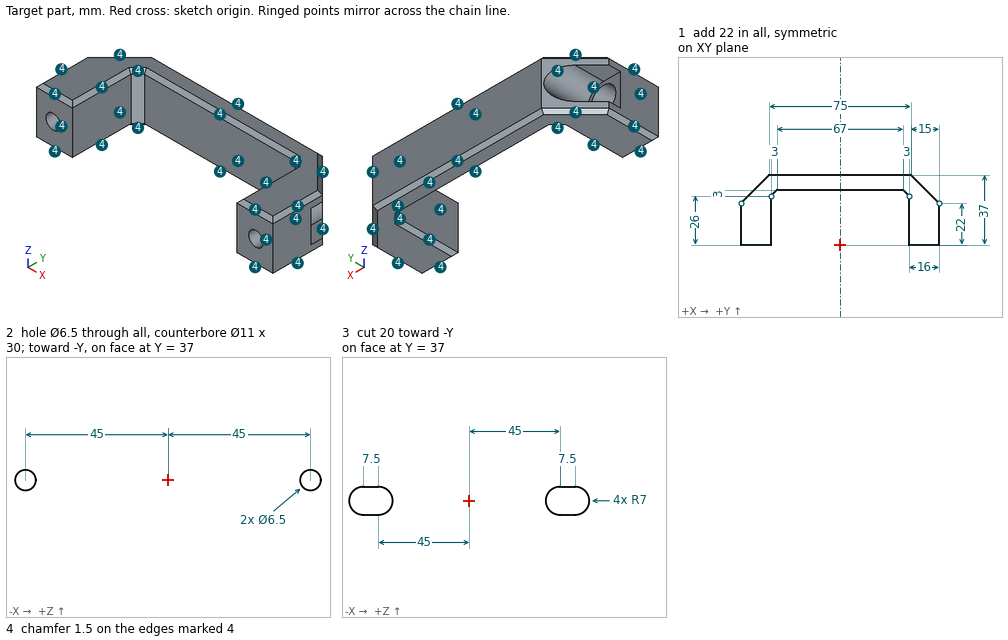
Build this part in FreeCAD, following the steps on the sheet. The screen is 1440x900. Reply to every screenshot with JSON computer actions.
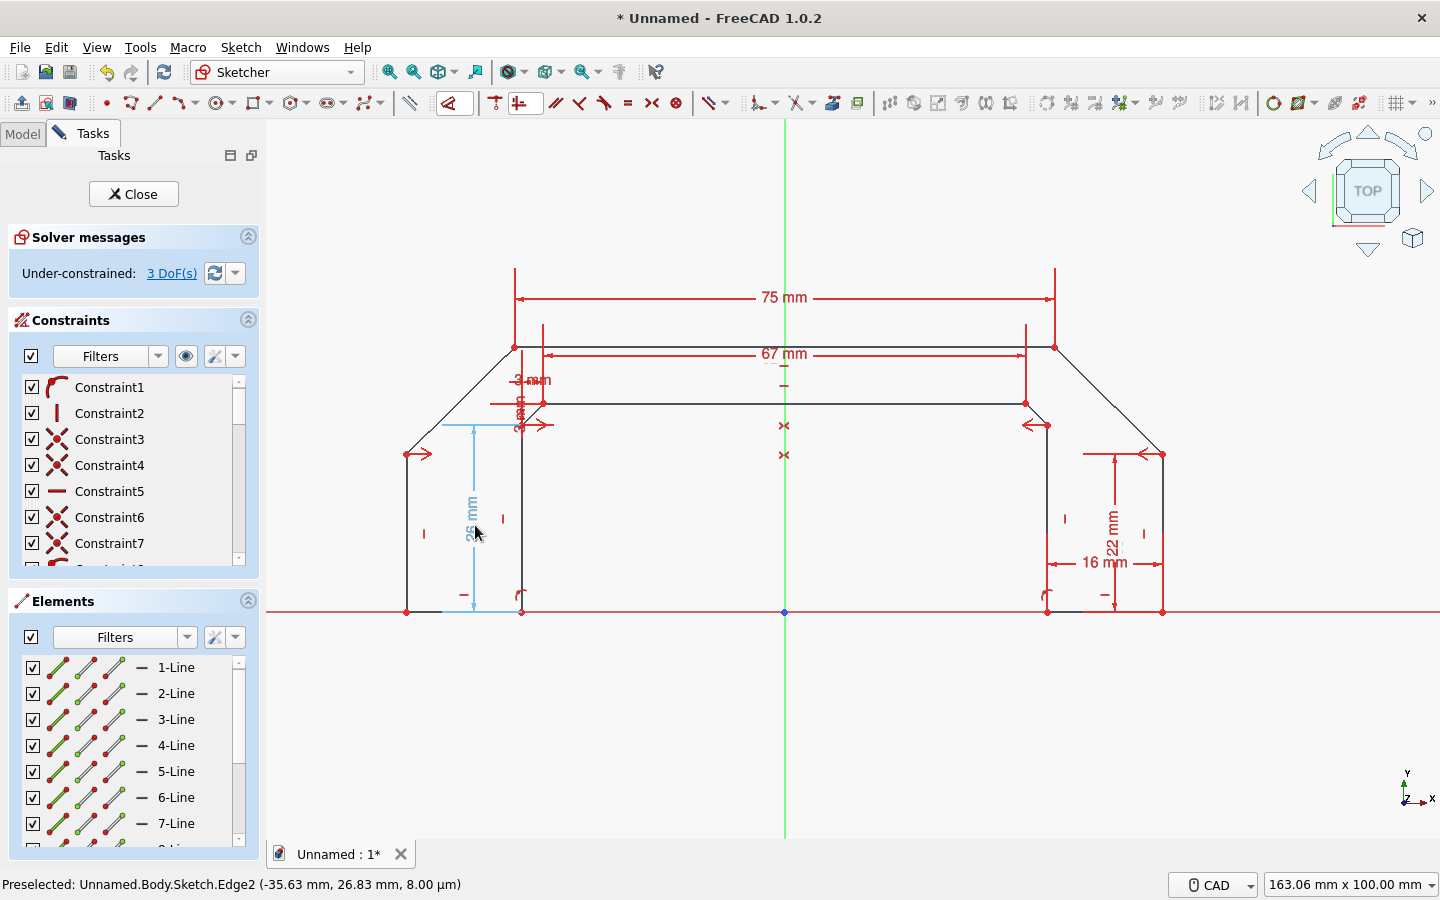
{"action": "scroll", "coordinate": [1032, 410], "scroll_direction": "up", "scroll_amount": 4}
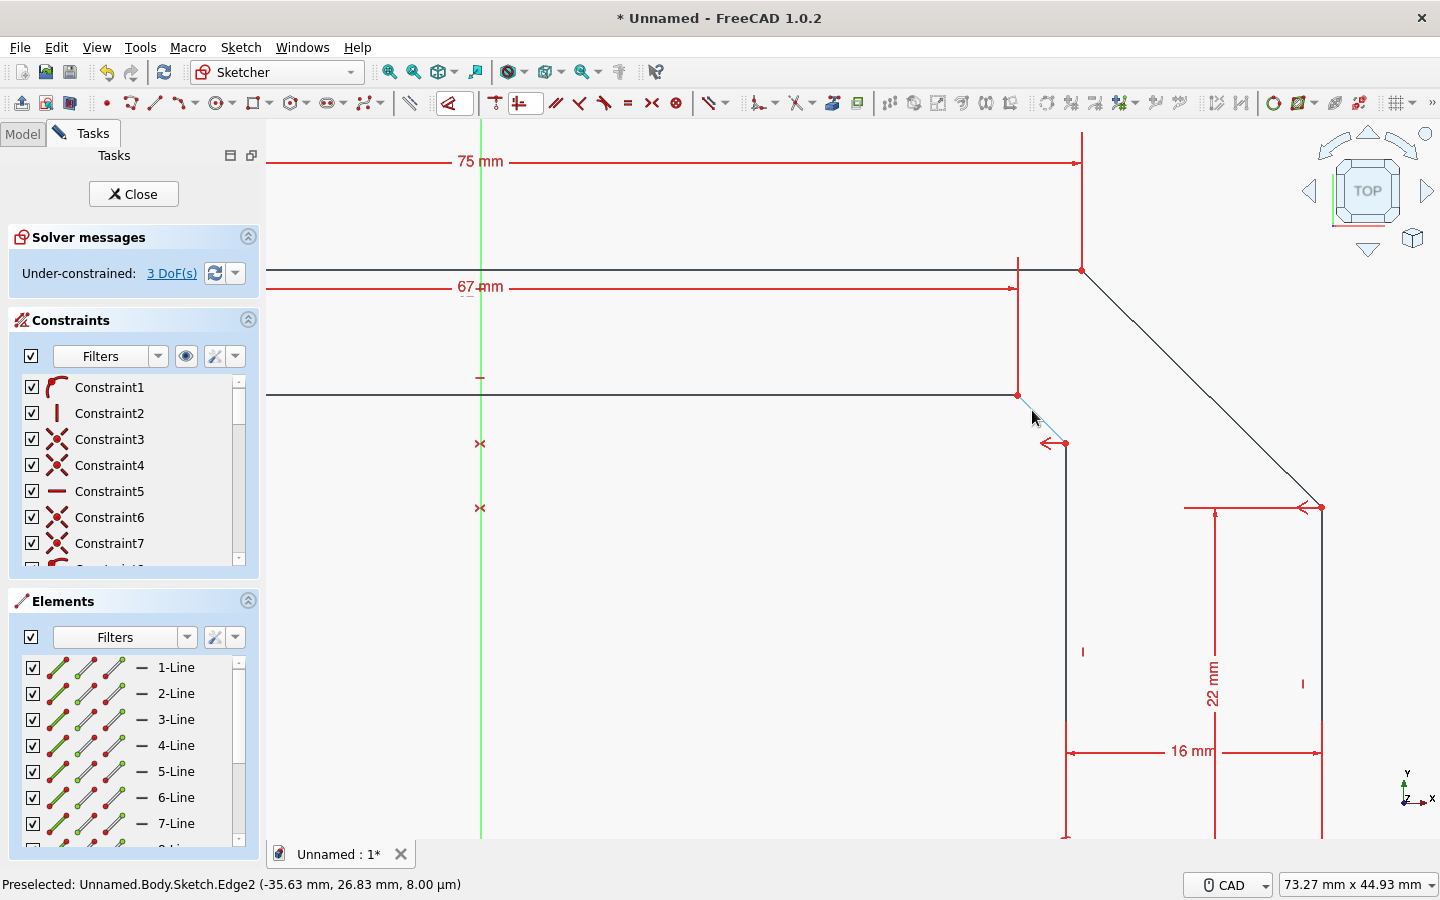
{"action": "left_click", "coordinate": [1032, 410]}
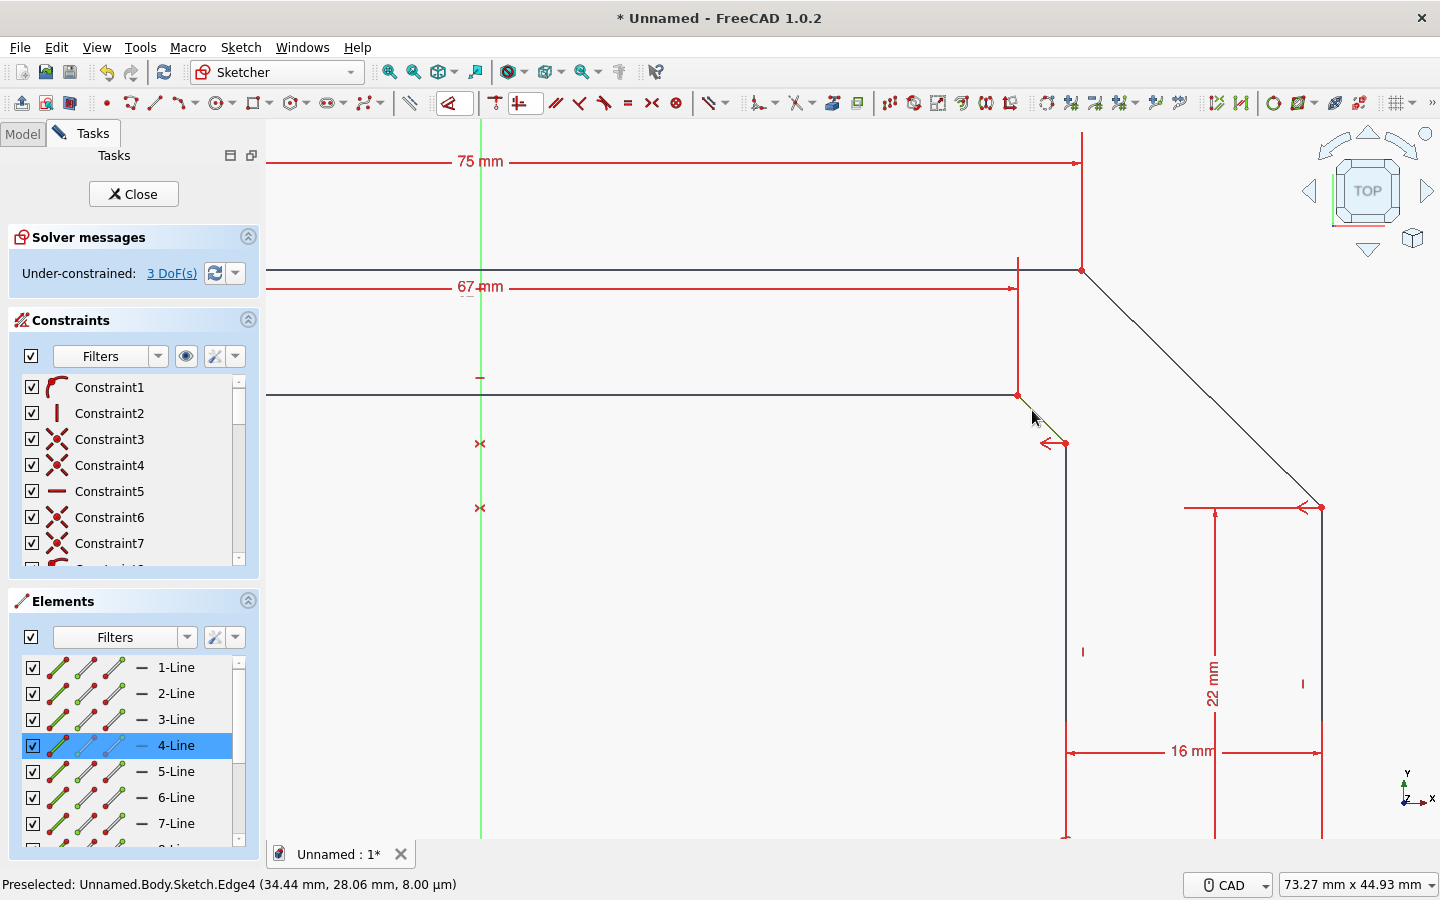
{"action": "key", "text": "l"}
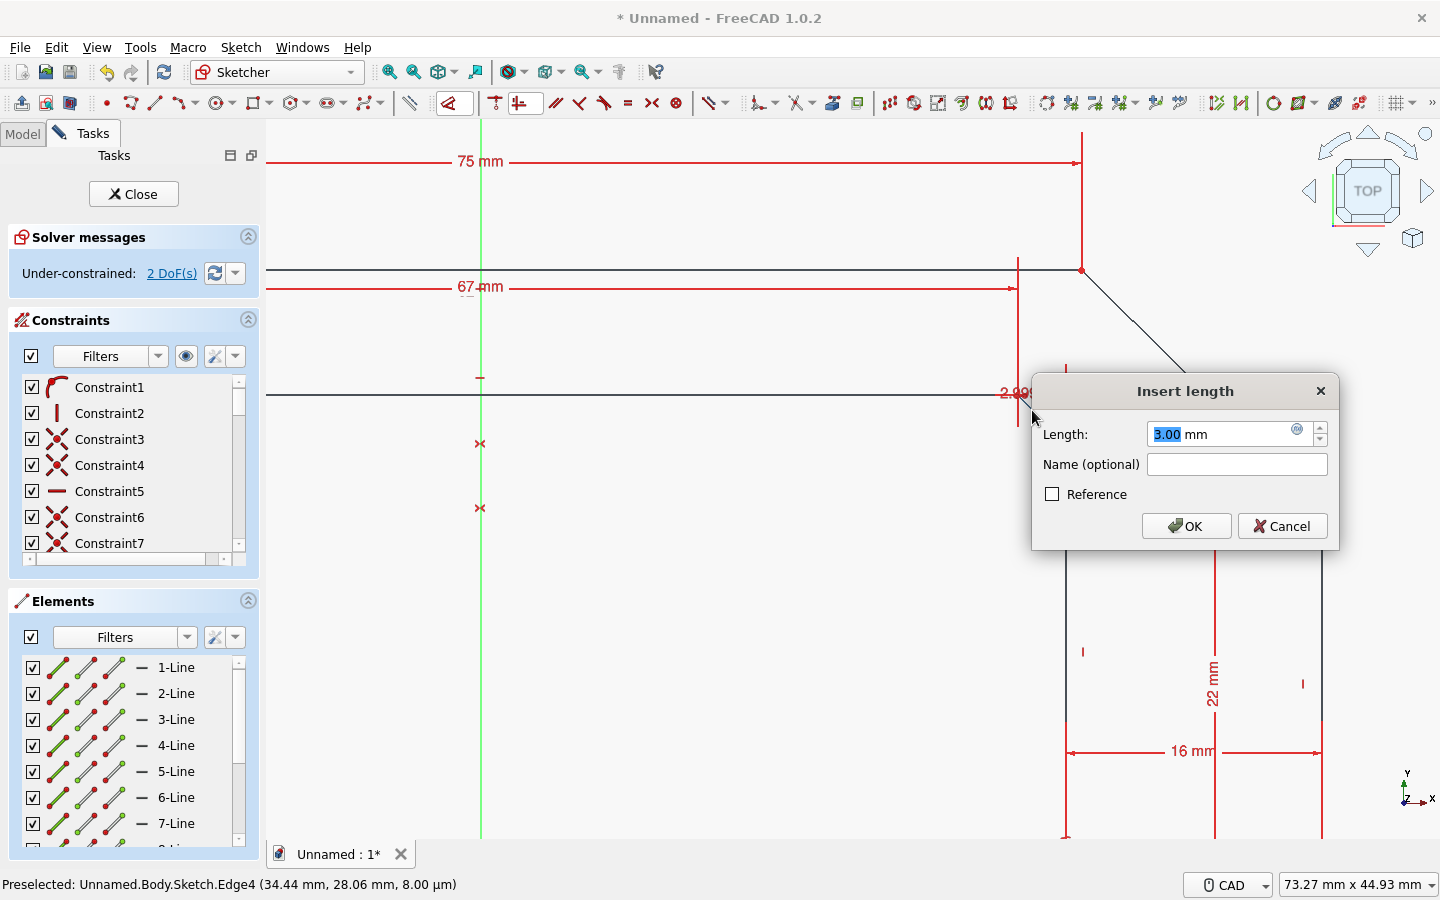
{"action": "type", "text": "3"}
{"action": "key", "text": "Return"}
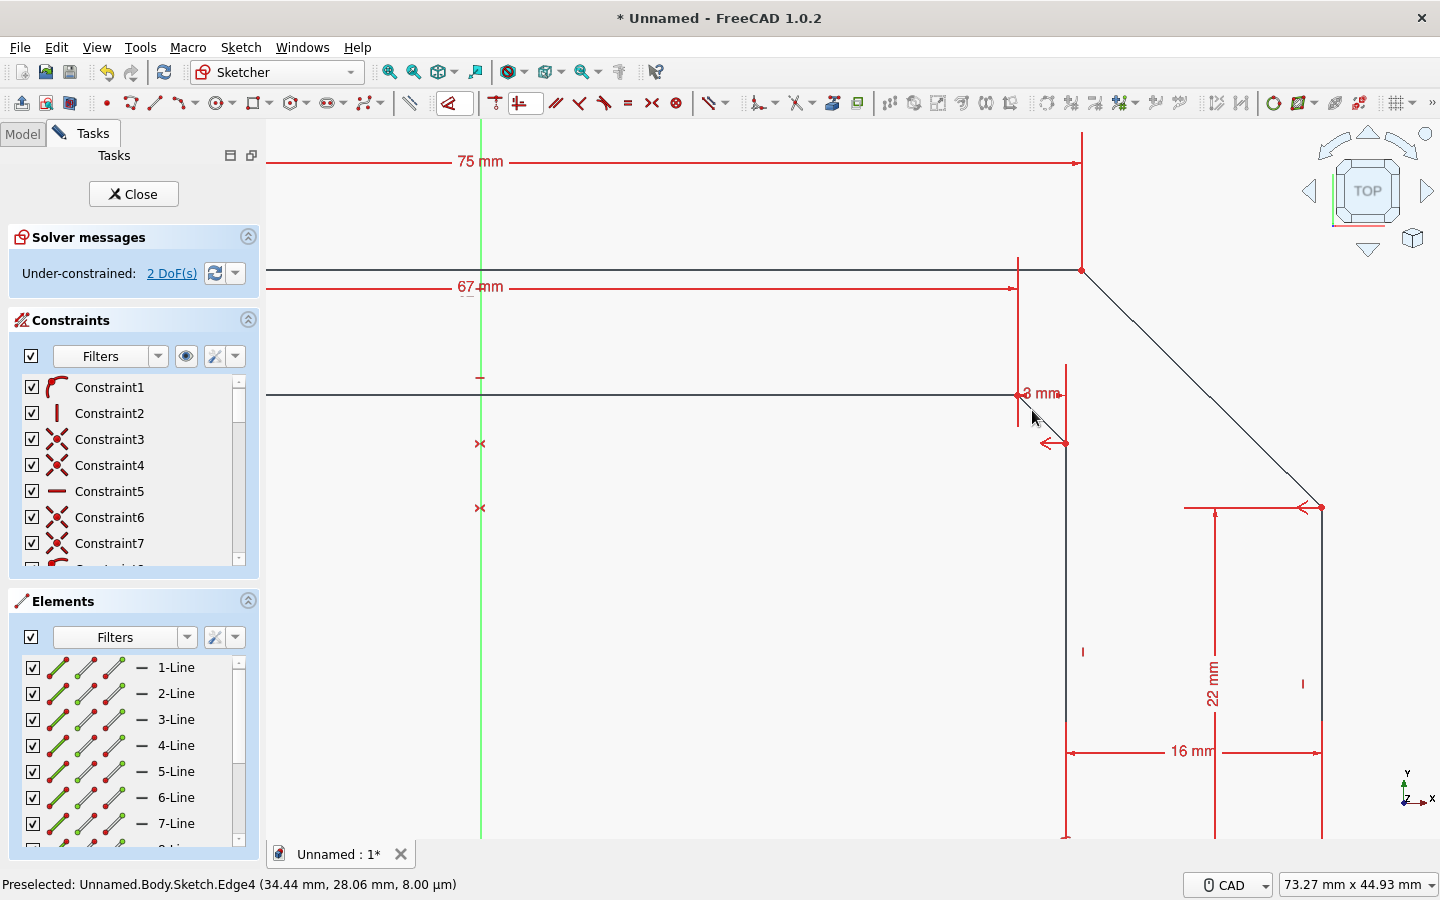
{"action": "left_click", "coordinate": [1082, 270]}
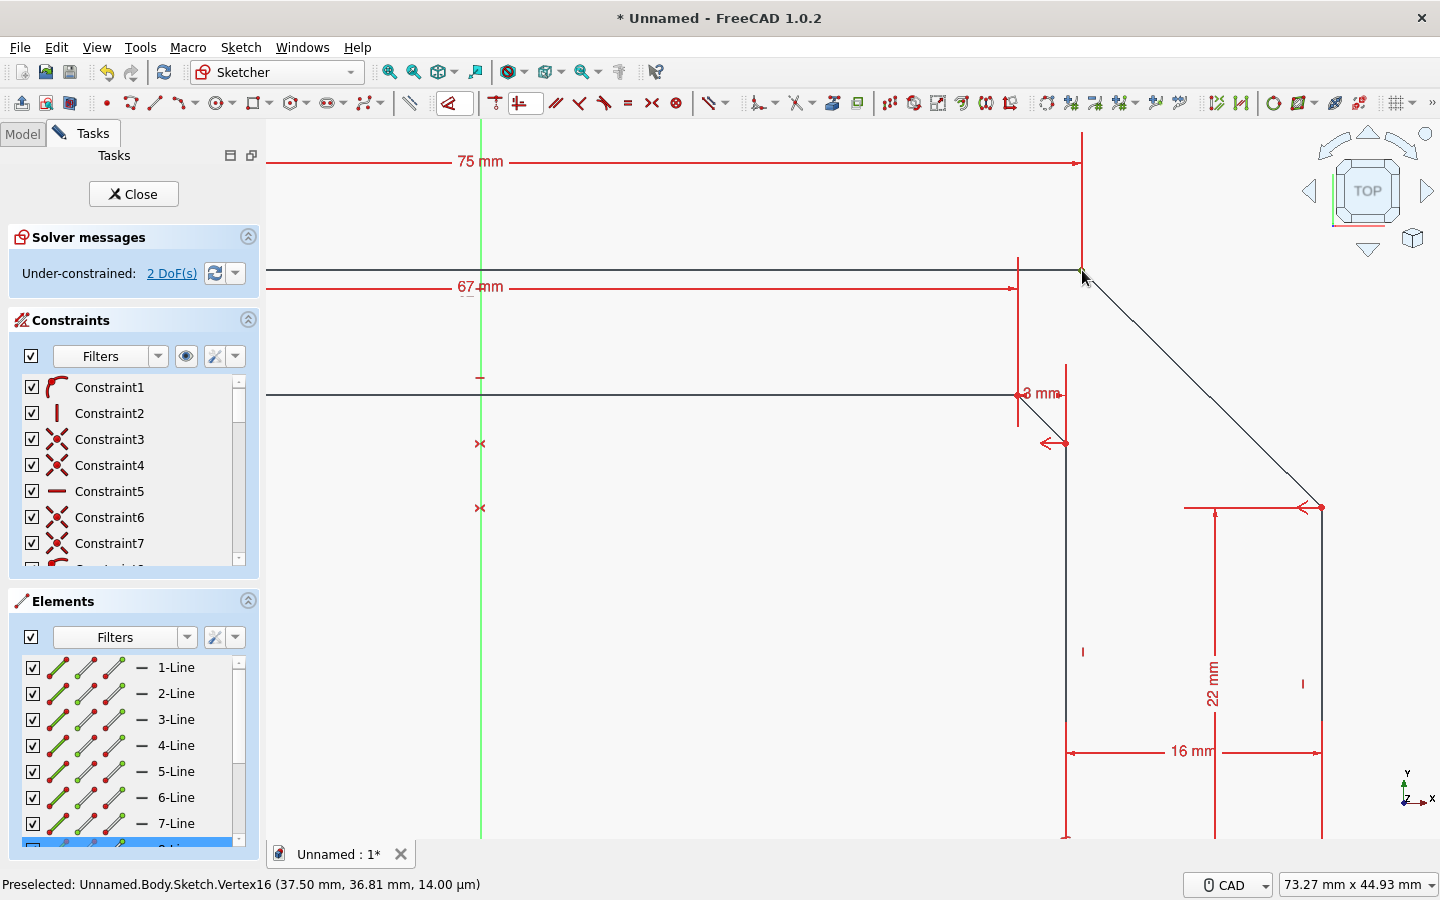
{"action": "key", "text": "i"}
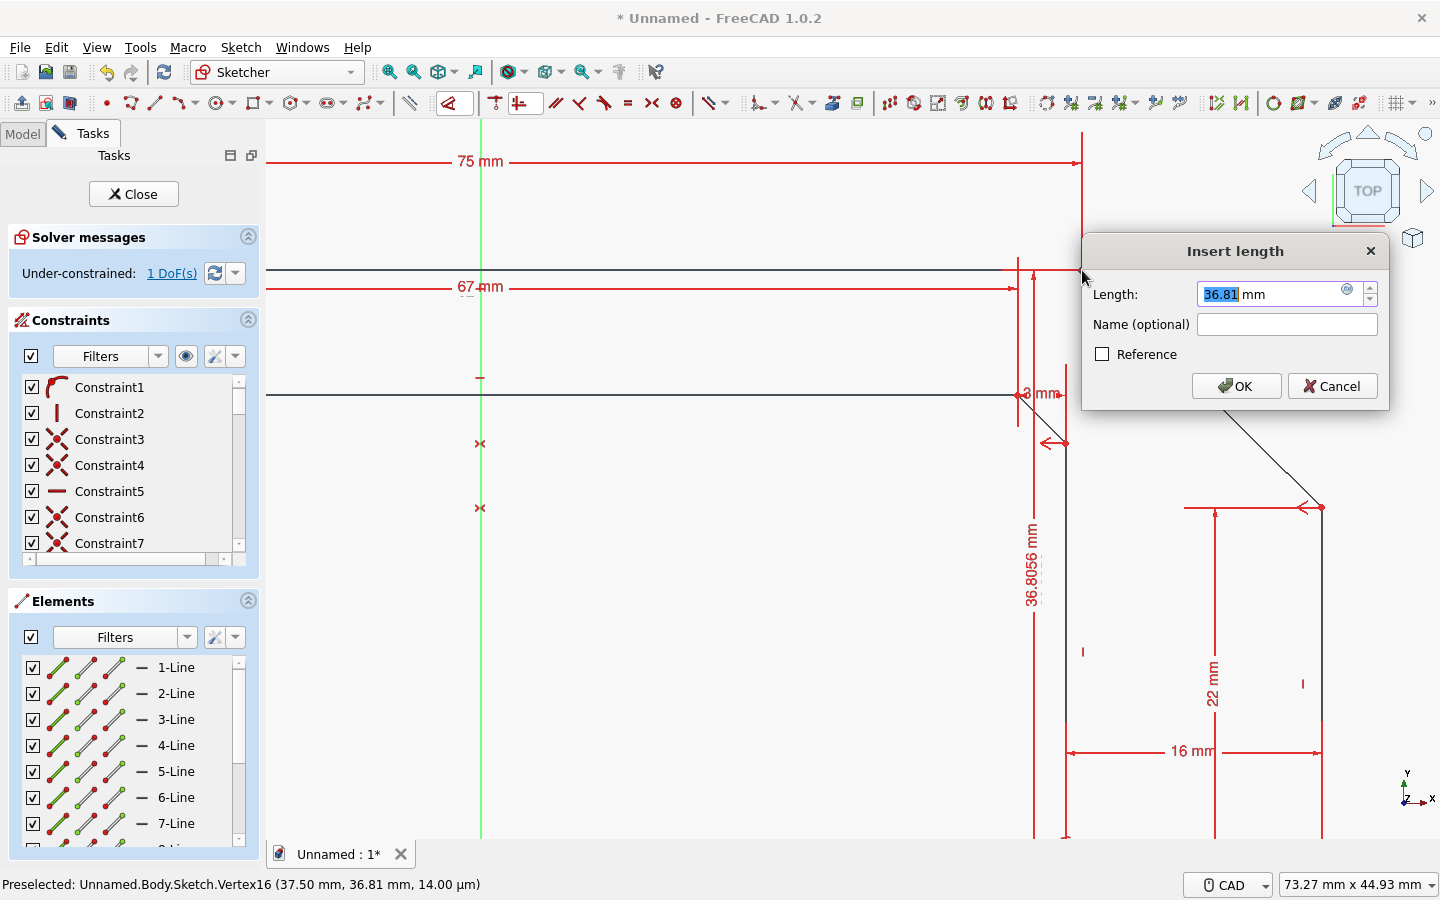
{"action": "type", "text": "37"}
{"action": "key", "text": "Return"}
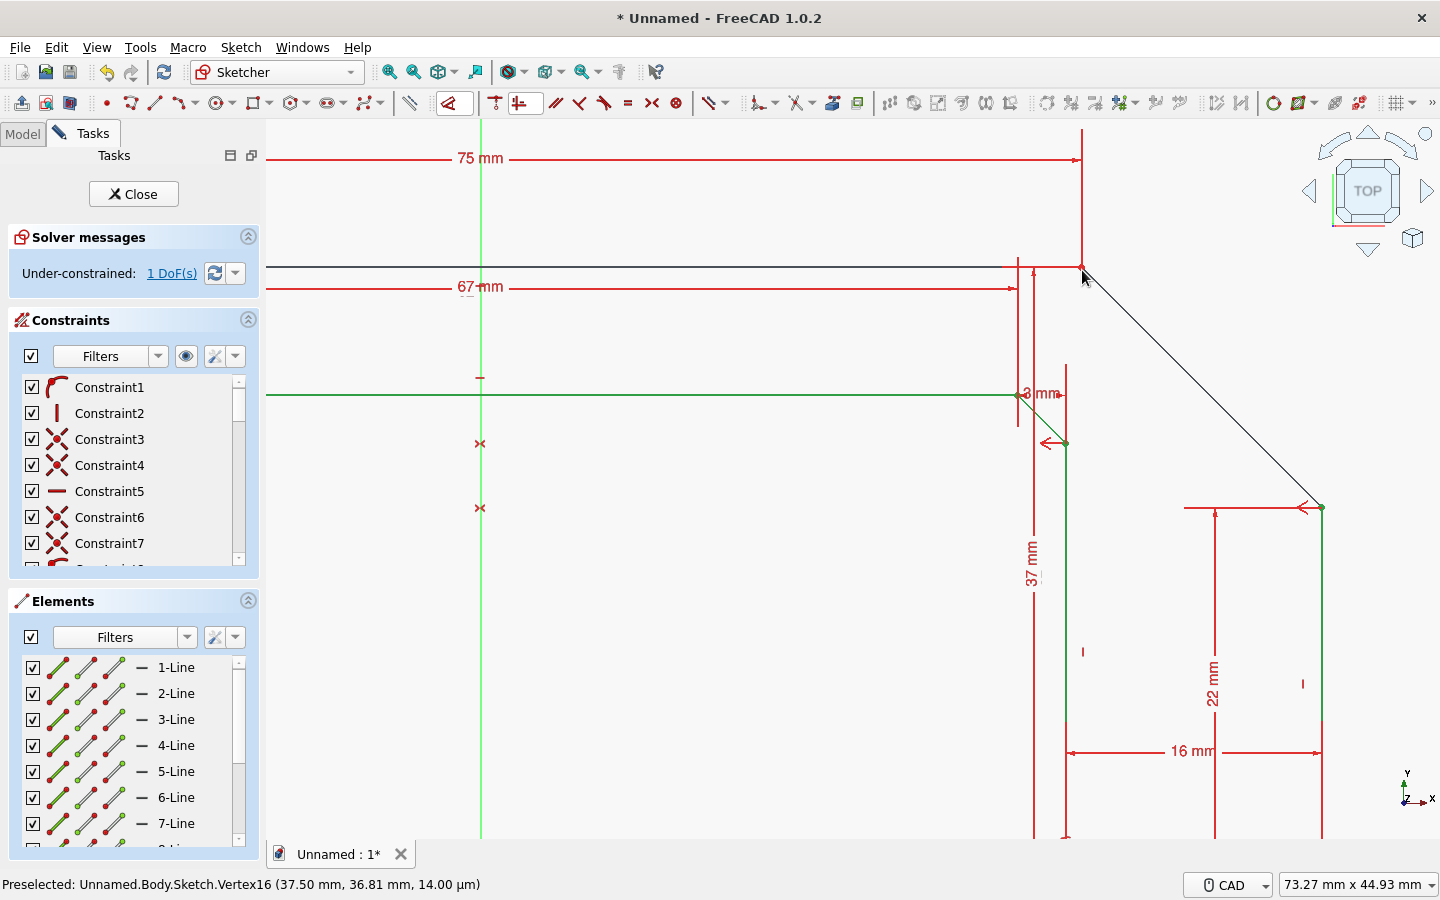
{"action": "left_click", "coordinate": [1250, 435]}